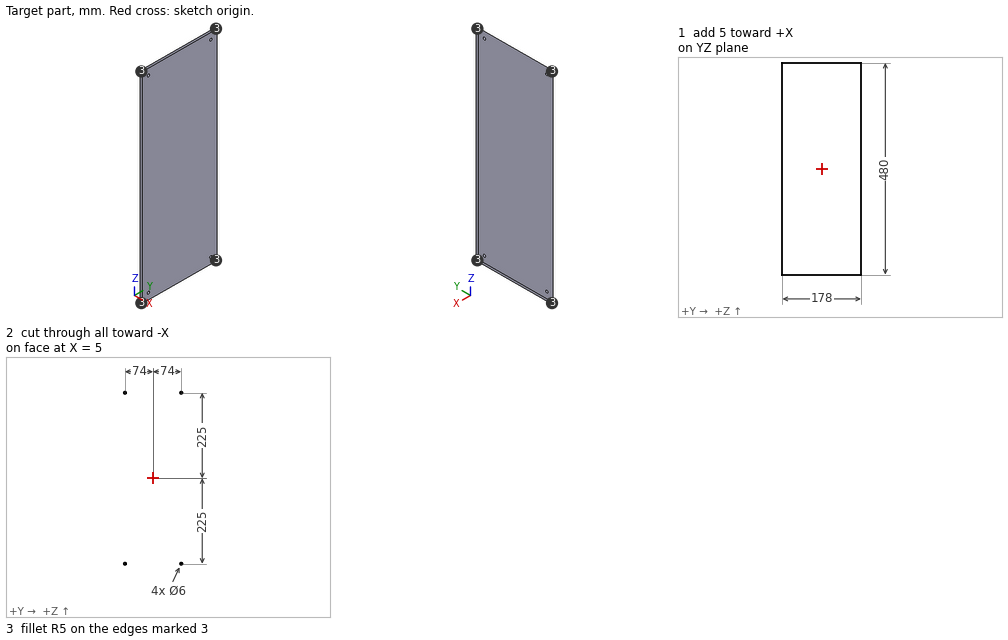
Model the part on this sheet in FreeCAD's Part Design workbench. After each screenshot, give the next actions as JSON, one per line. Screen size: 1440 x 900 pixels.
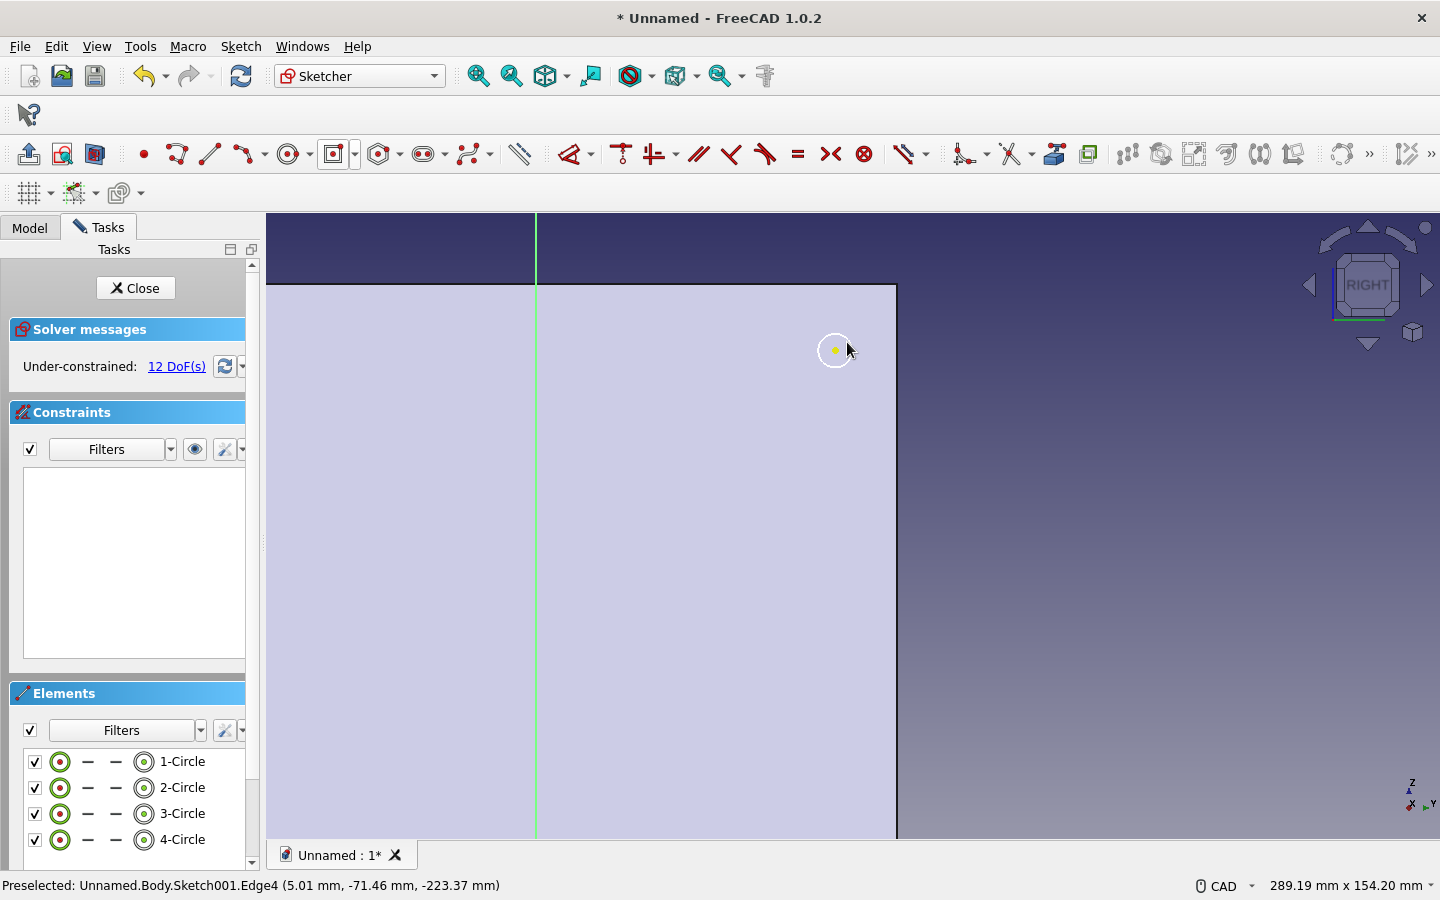
{"action": "left_click", "coordinate": [847, 339]}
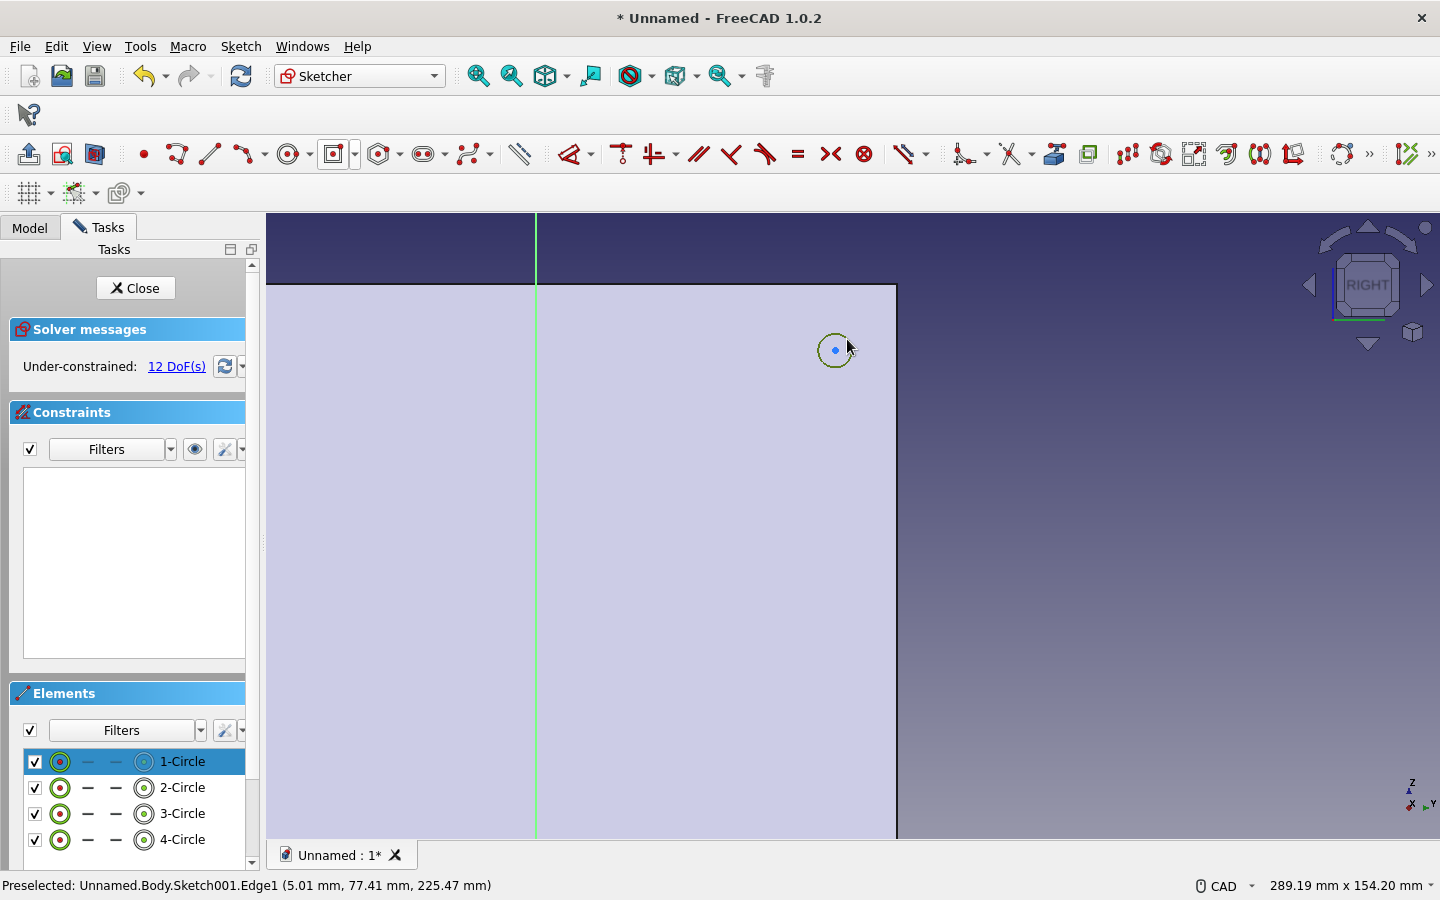
{"action": "scroll", "coordinate": [847, 341], "scroll_direction": "down", "scroll_amount": 8}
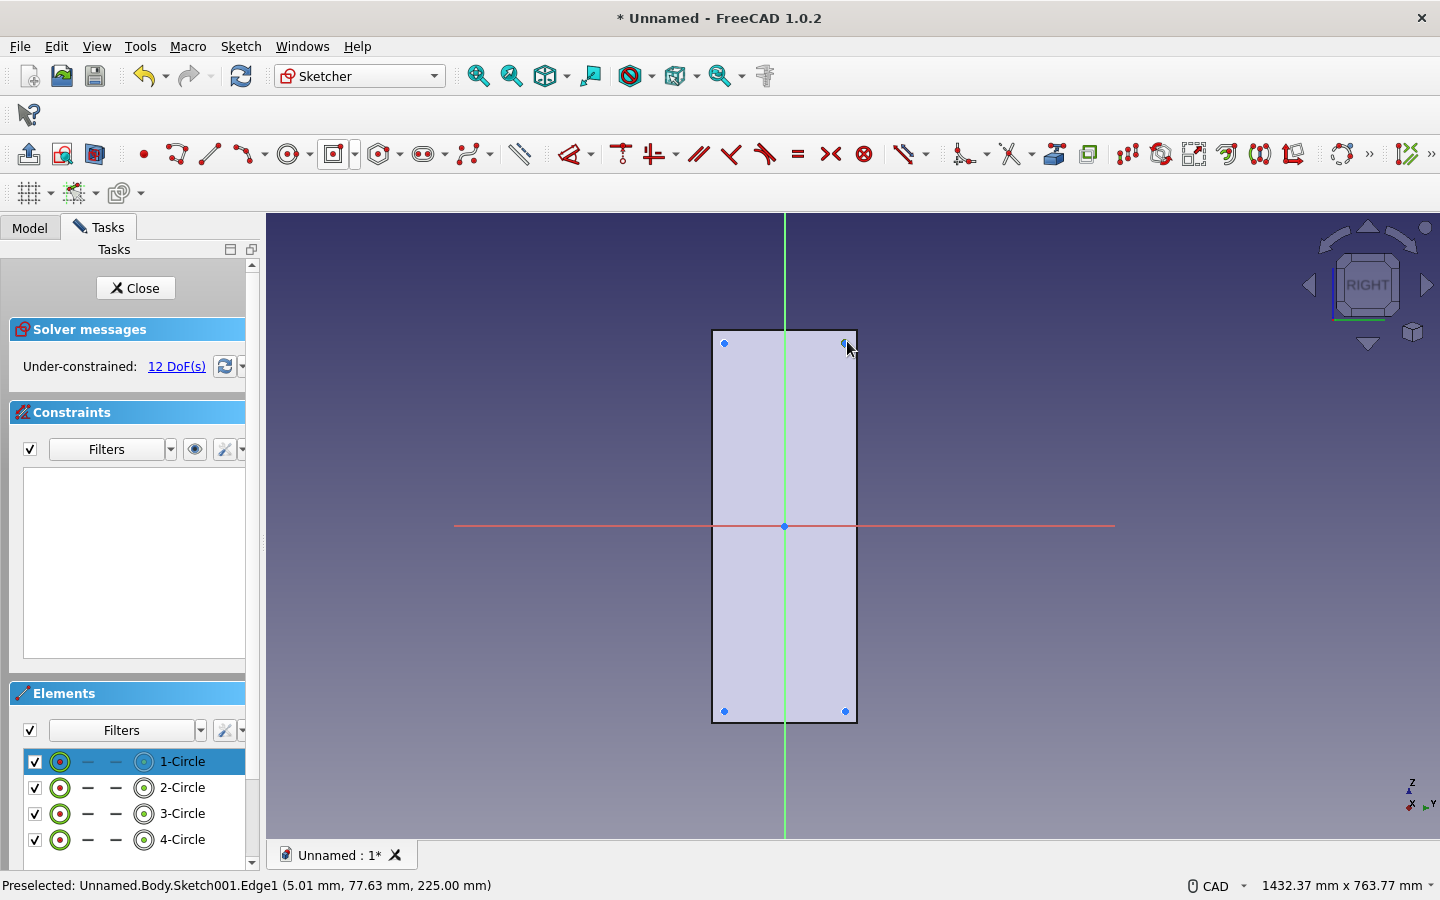
{"action": "scroll", "coordinate": [847, 709], "scroll_direction": "up", "scroll_amount": 8}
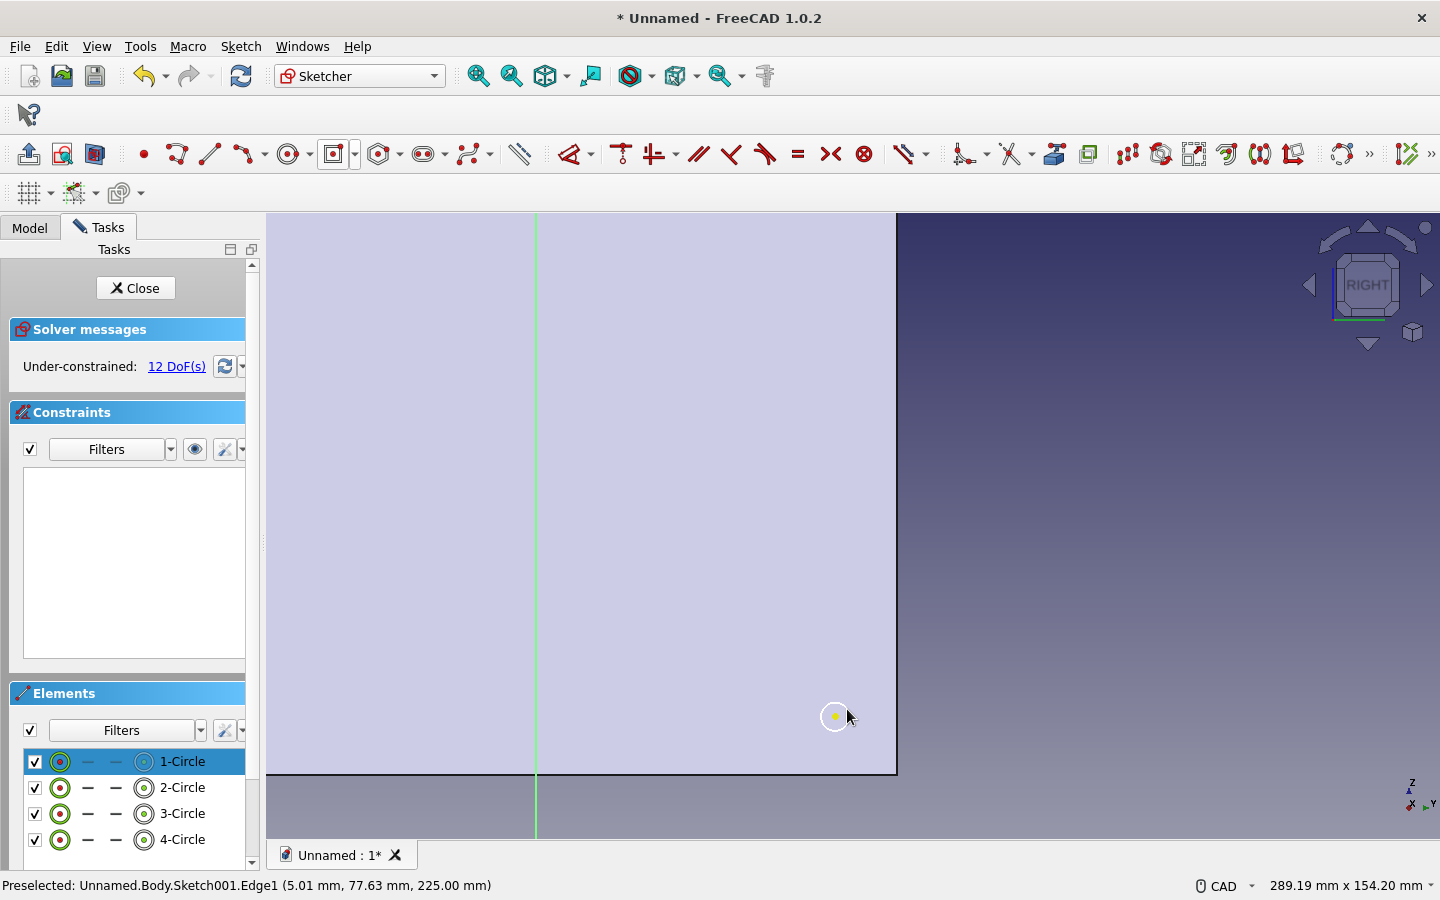
{"action": "left_click", "coordinate": [845, 707]}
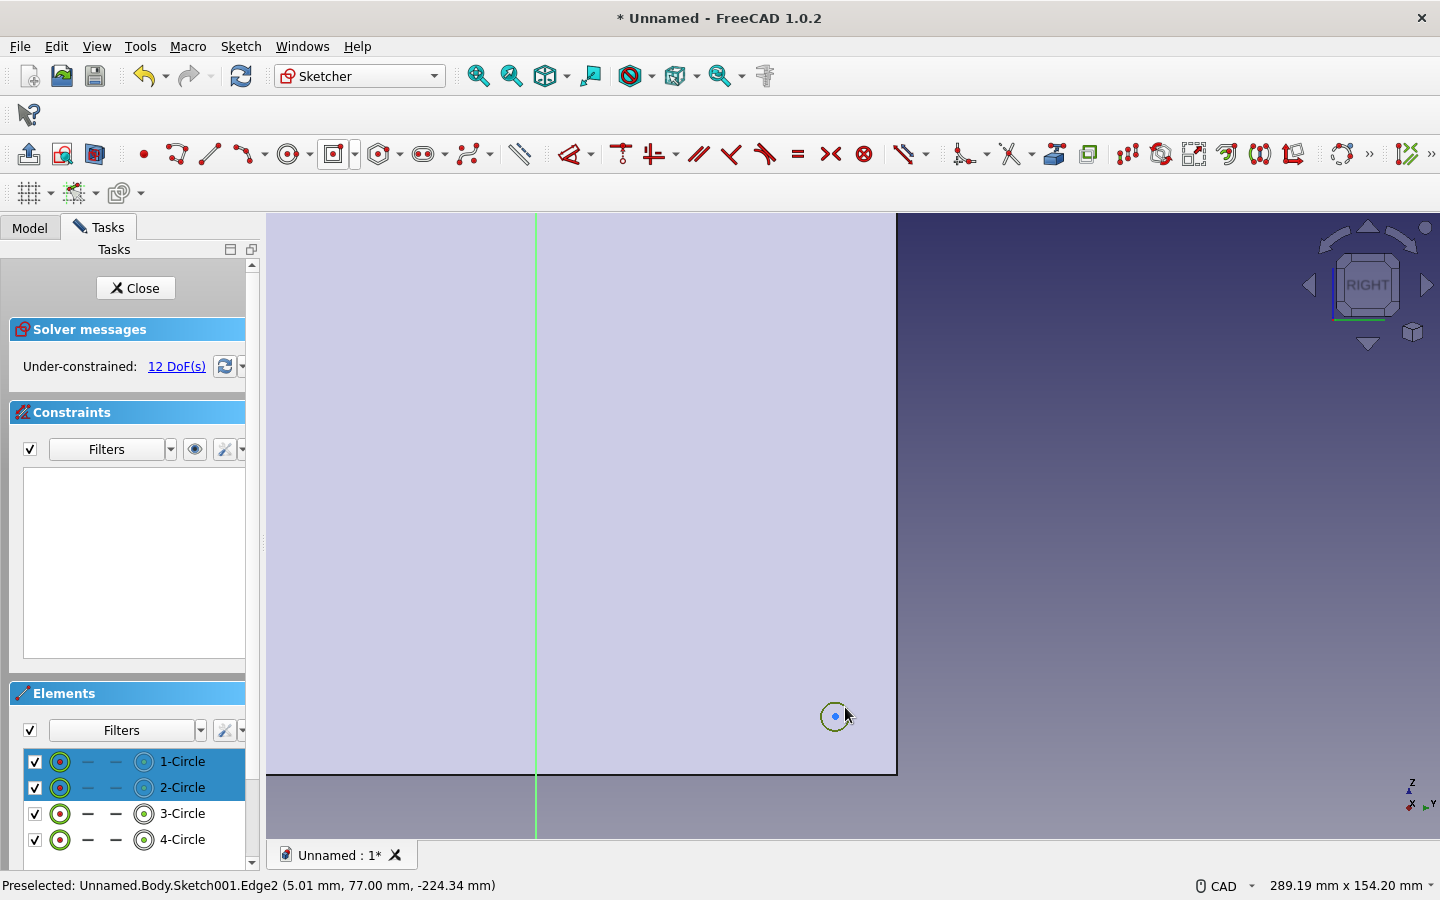
{"action": "scroll", "coordinate": [847, 709], "scroll_direction": "down", "scroll_amount": 8}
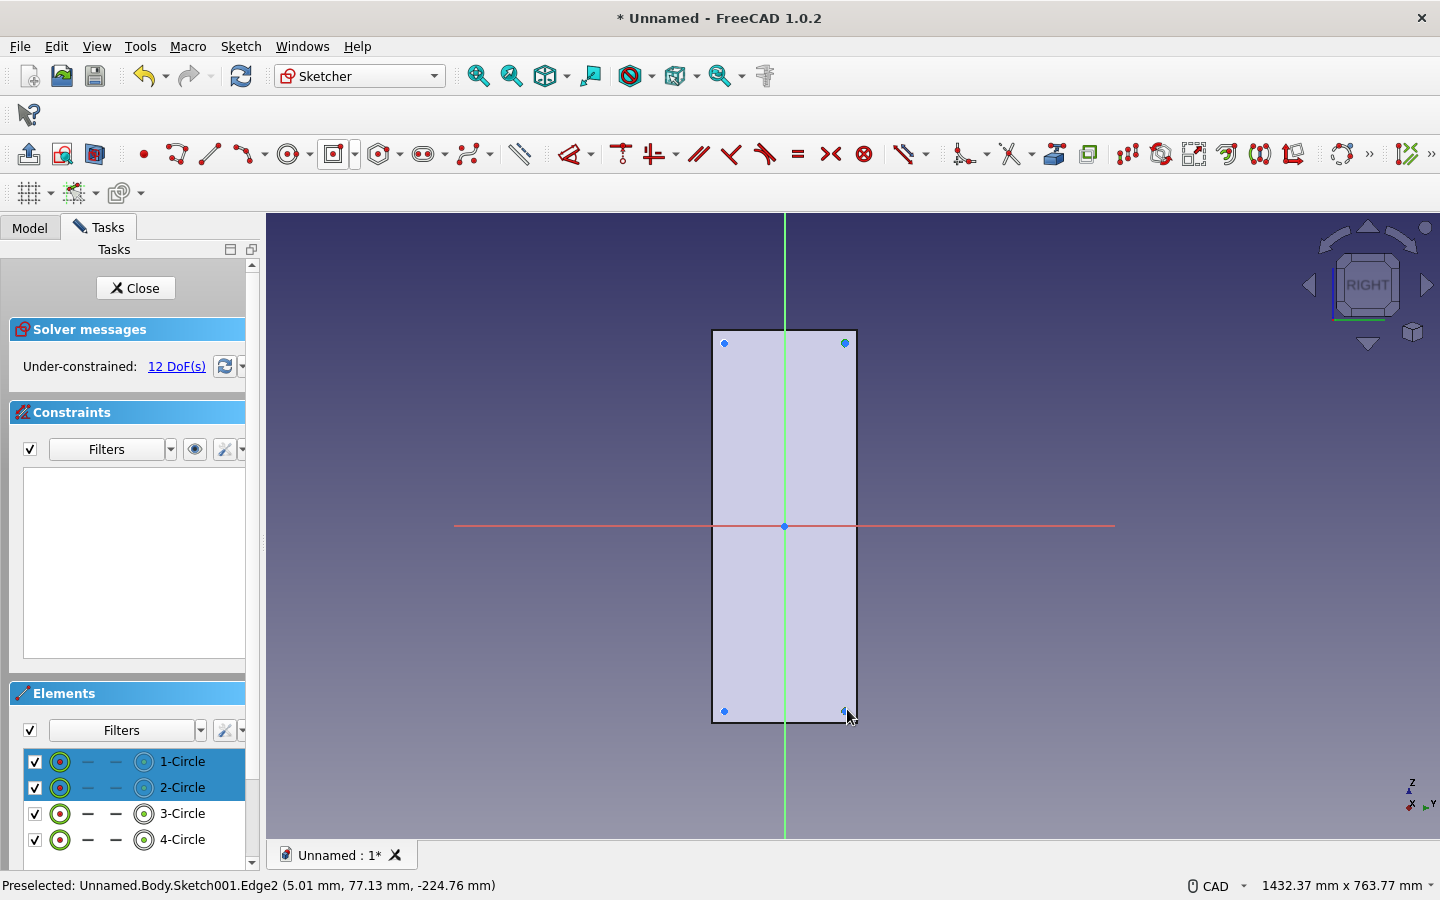
{"action": "scroll", "coordinate": [726, 341], "scroll_direction": "up", "scroll_amount": 8}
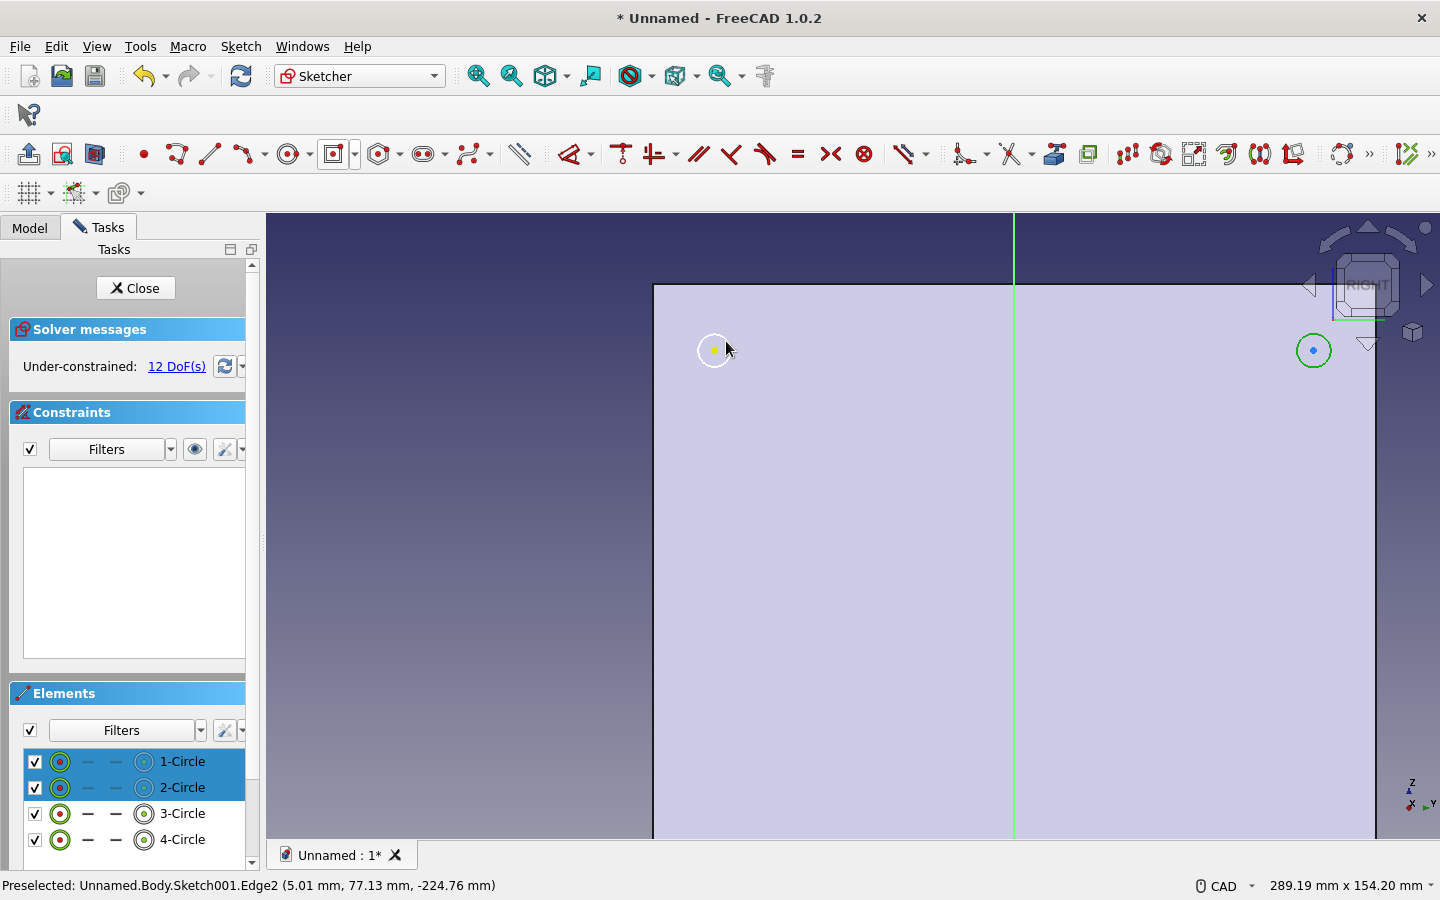
{"action": "left_click", "coordinate": [726, 339]}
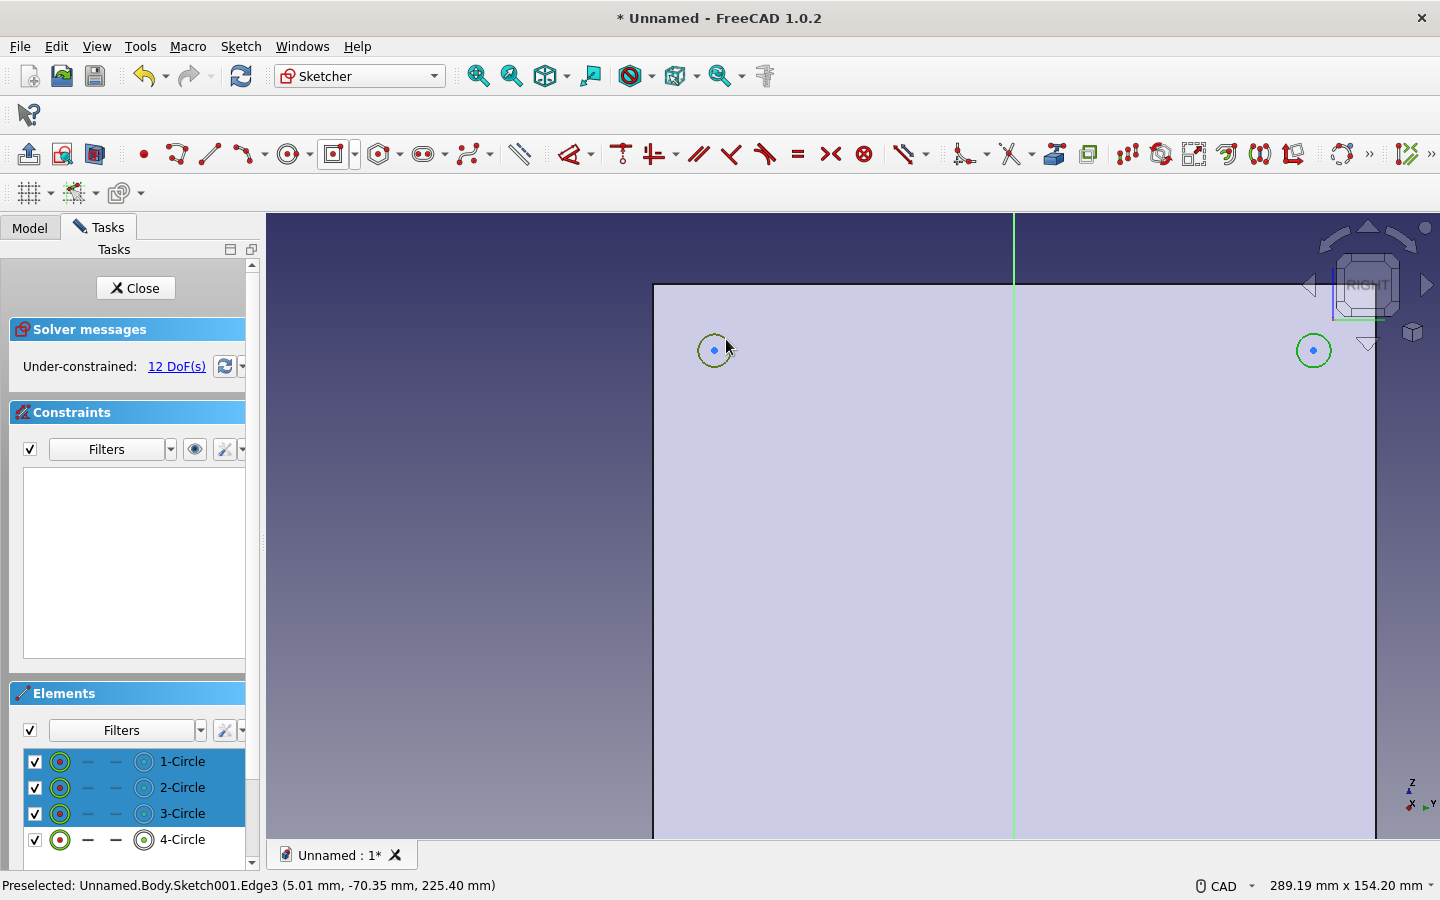
{"action": "scroll", "coordinate": [726, 341], "scroll_direction": "down", "scroll_amount": 8}